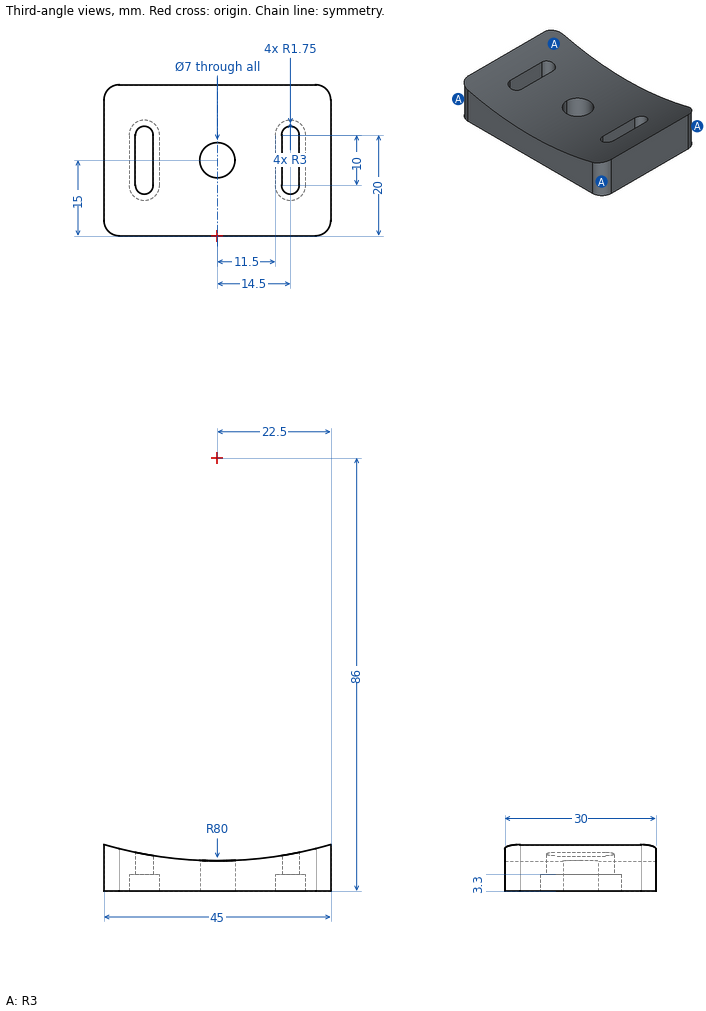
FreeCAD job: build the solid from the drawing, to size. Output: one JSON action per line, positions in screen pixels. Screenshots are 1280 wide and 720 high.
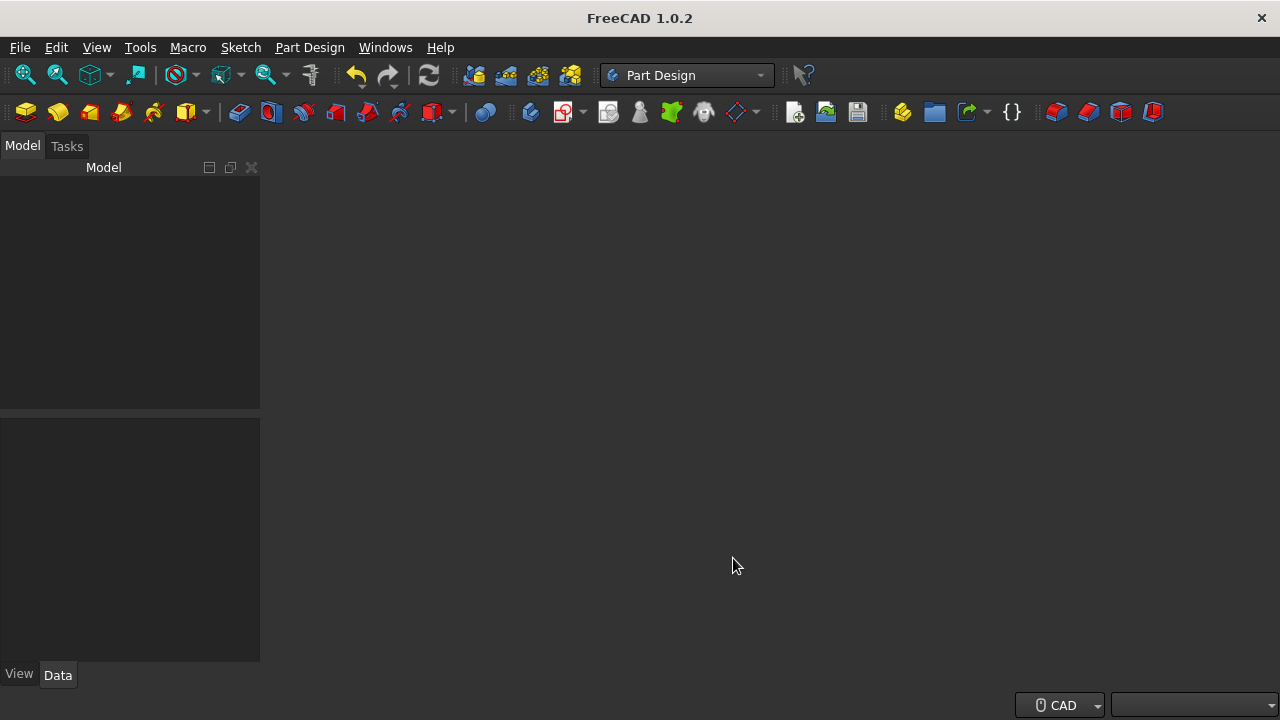
{"action": "key", "text": "ctrl+n"}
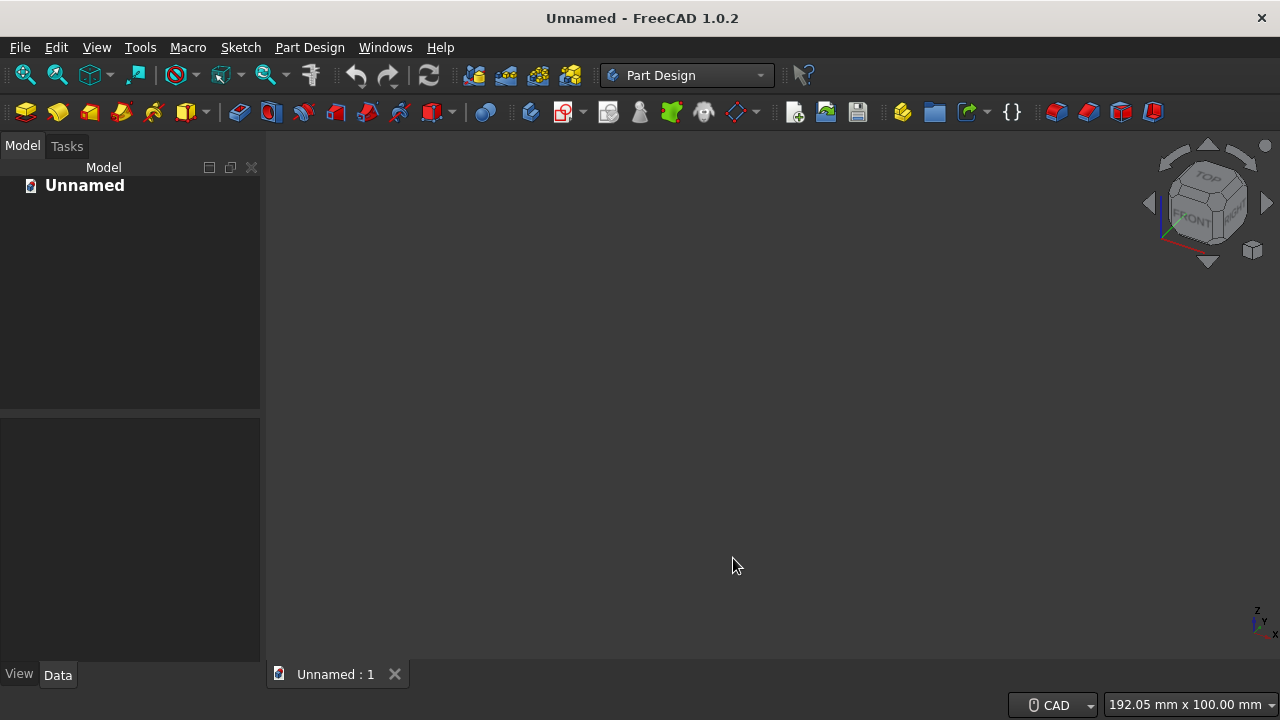
{"action": "left_click", "coordinate": [564, 112]}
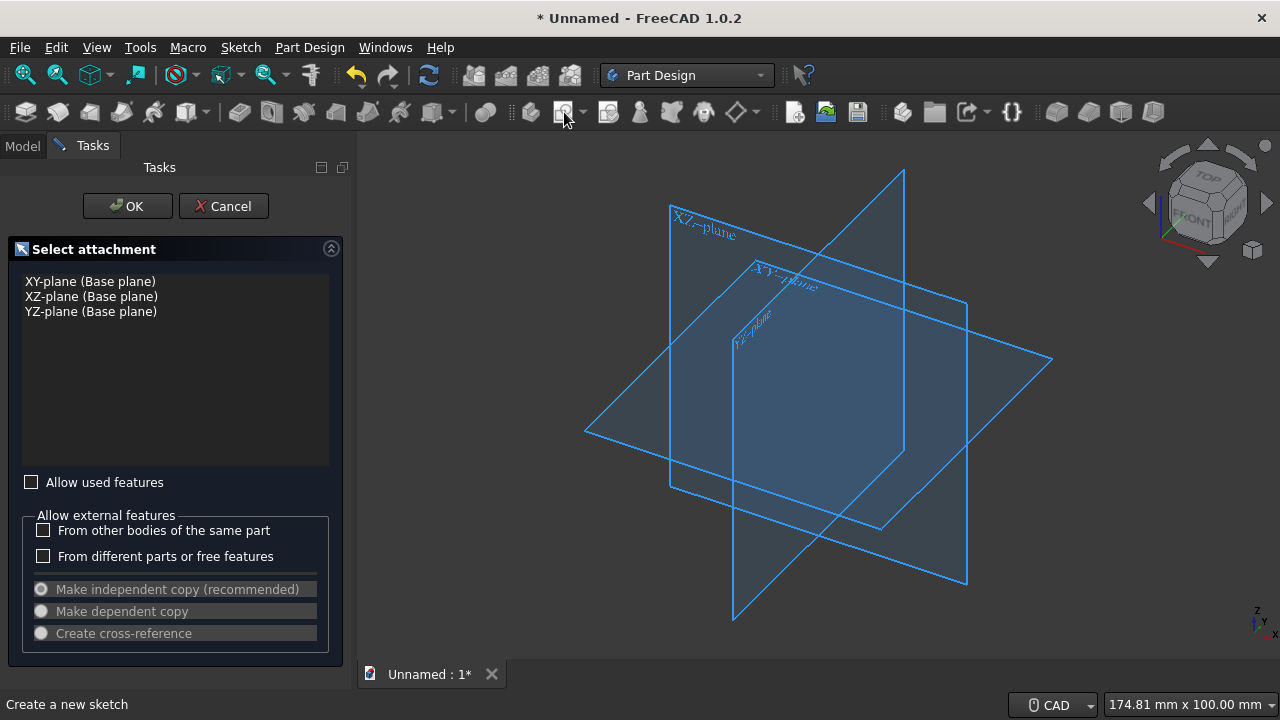
{"action": "left_click", "coordinate": [82, 296]}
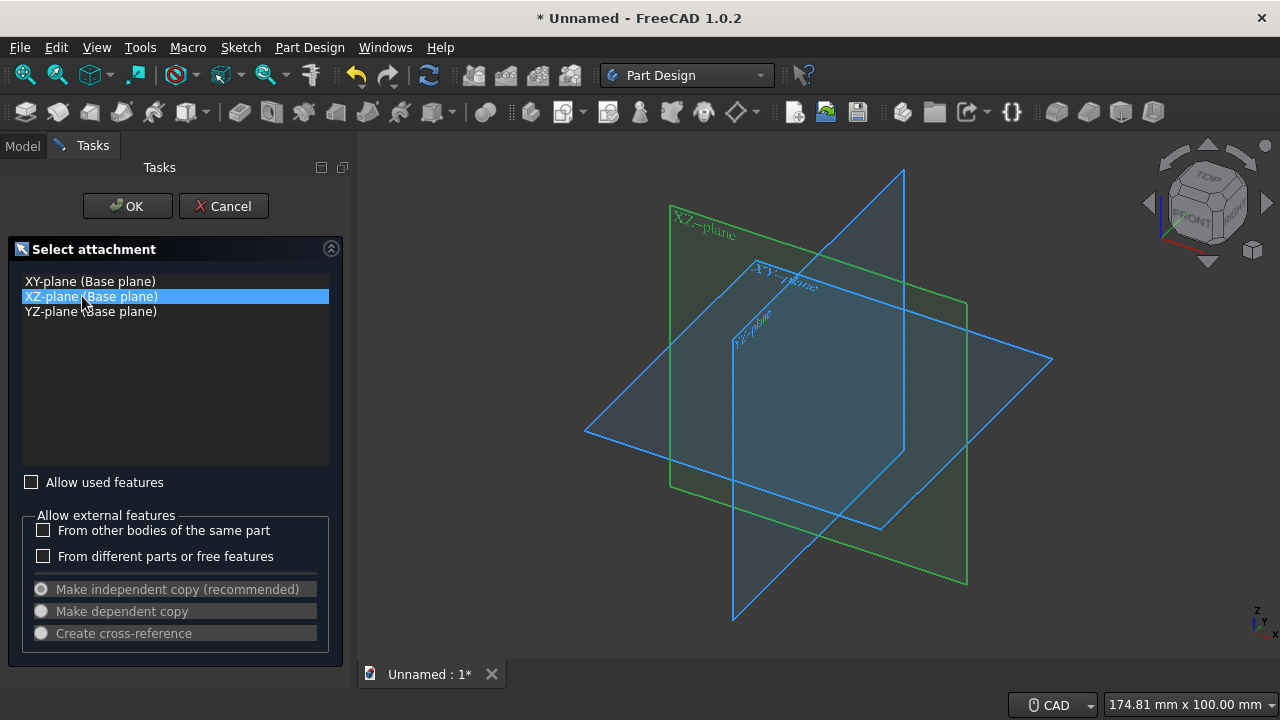
{"action": "left_click", "coordinate": [128, 206]}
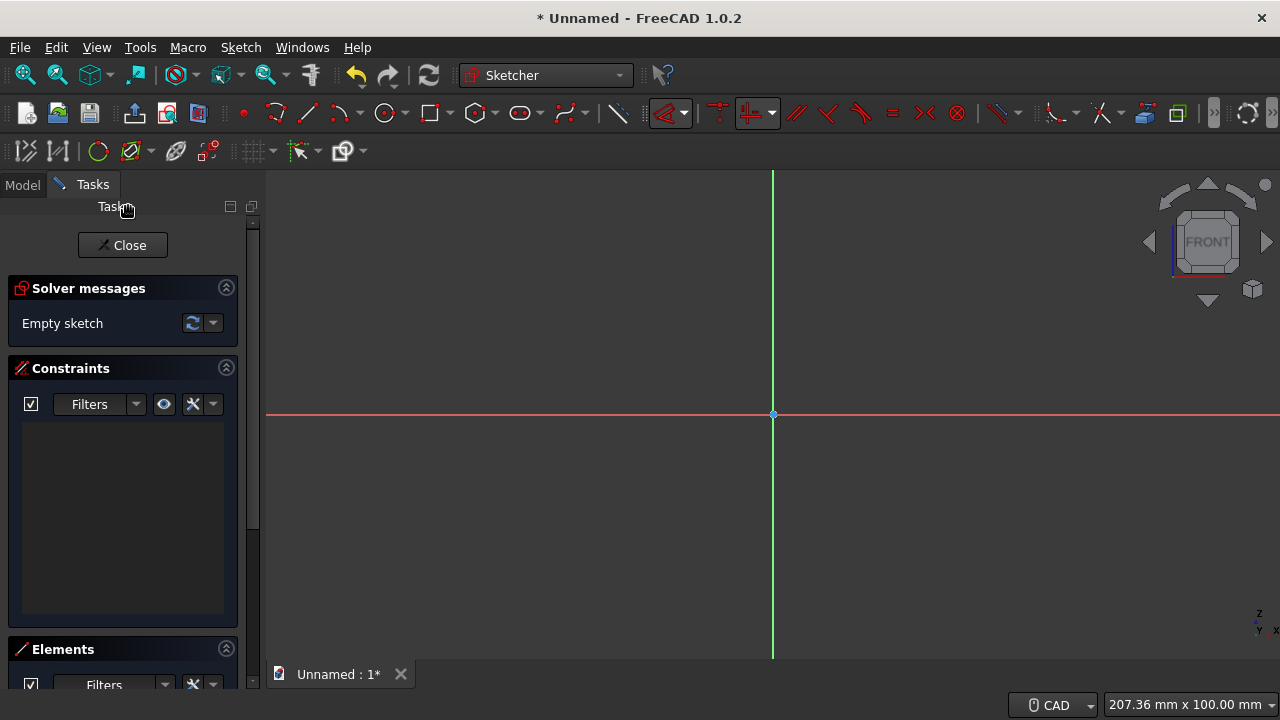
{"action": "scroll", "coordinate": [621, 198], "scroll_direction": "down", "scroll_amount": 3}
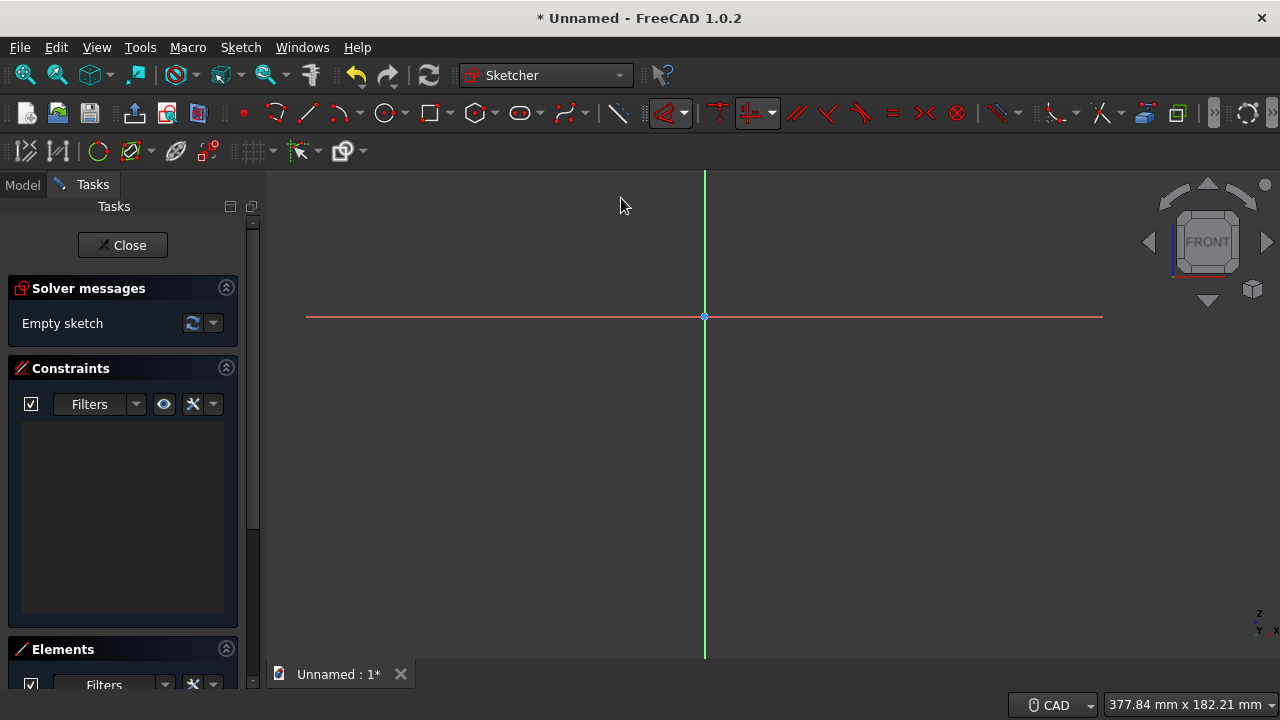
{"action": "left_click", "coordinate": [276, 114]}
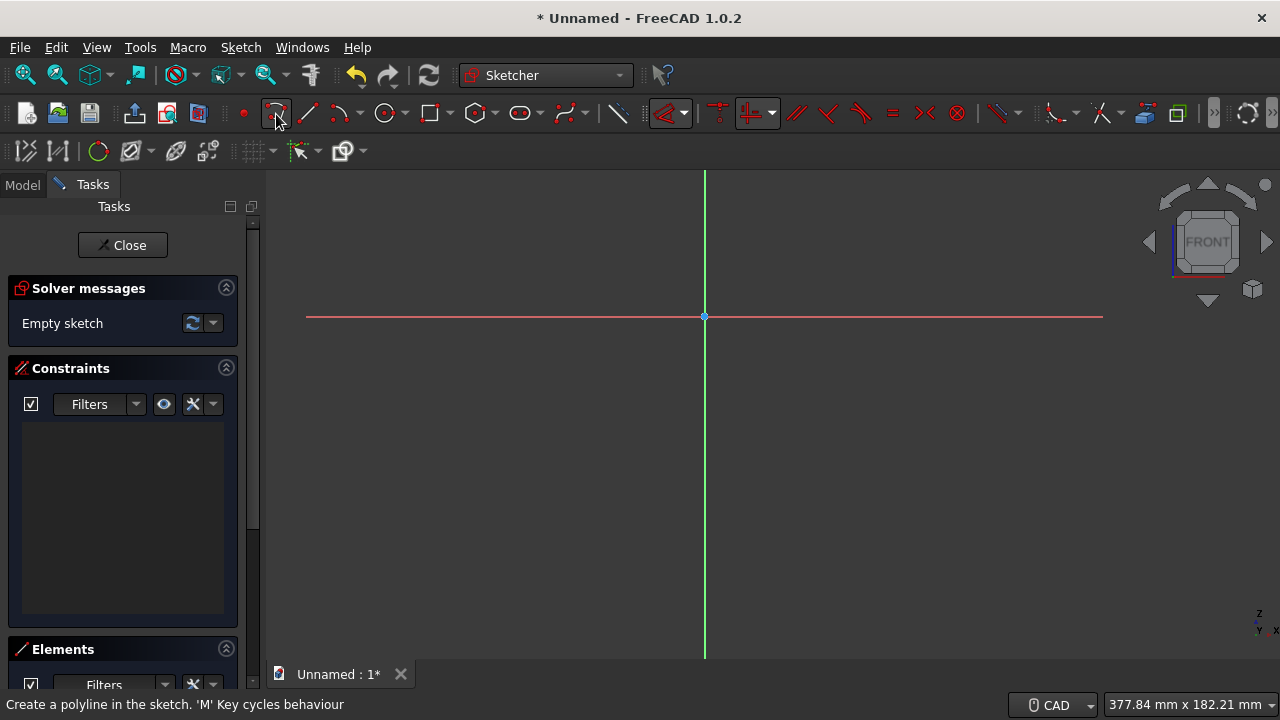
{"action": "left_click", "coordinate": [765, 523]}
{"action": "left_click", "coordinate": [765, 548]}
{"action": "left_click", "coordinate": [644, 548]}
{"action": "left_click", "coordinate": [644, 523]}
{"action": "right_click", "coordinate": [644, 523]}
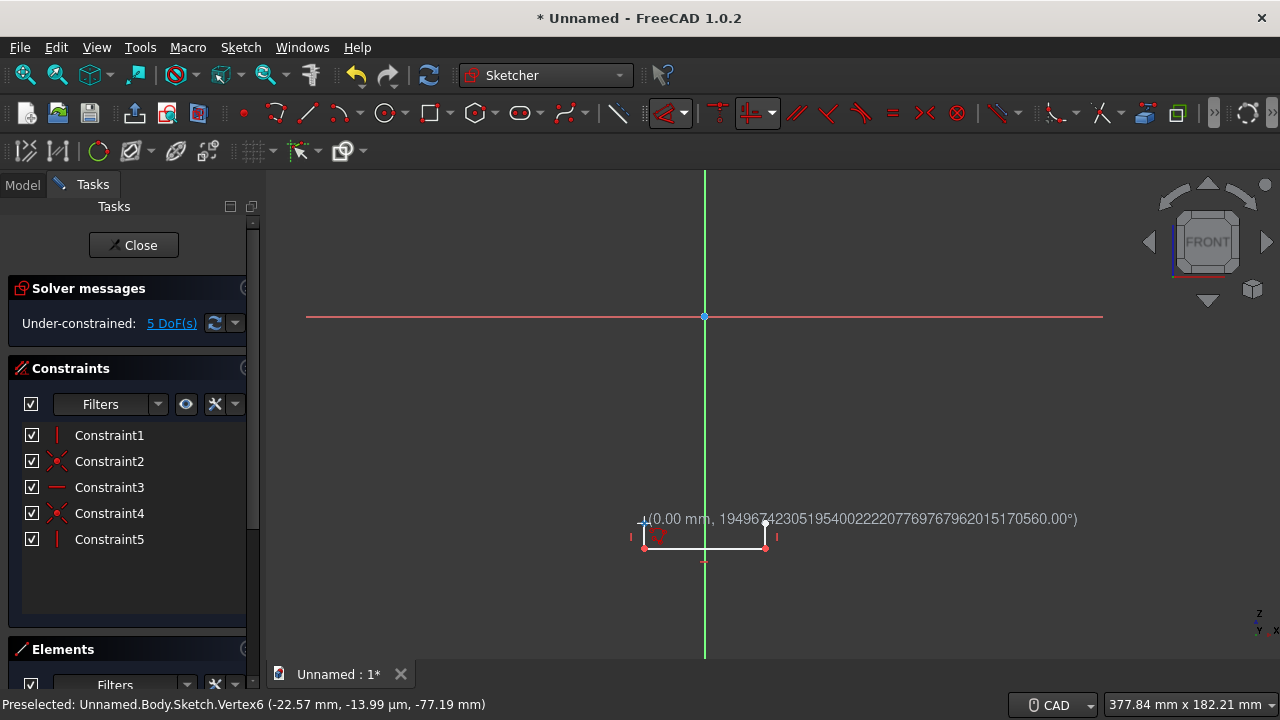
{"action": "key", "text": "g 3 a"}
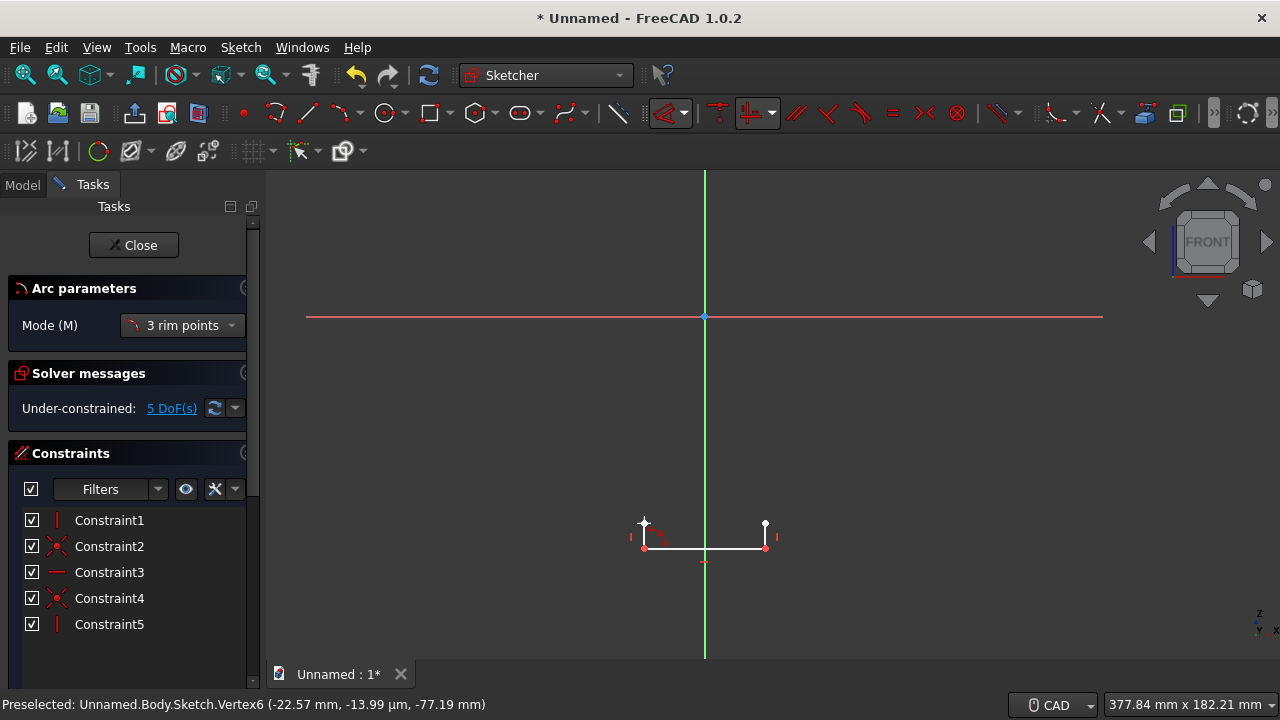
{"action": "scroll", "coordinate": [644, 523], "scroll_direction": "up", "scroll_amount": 2}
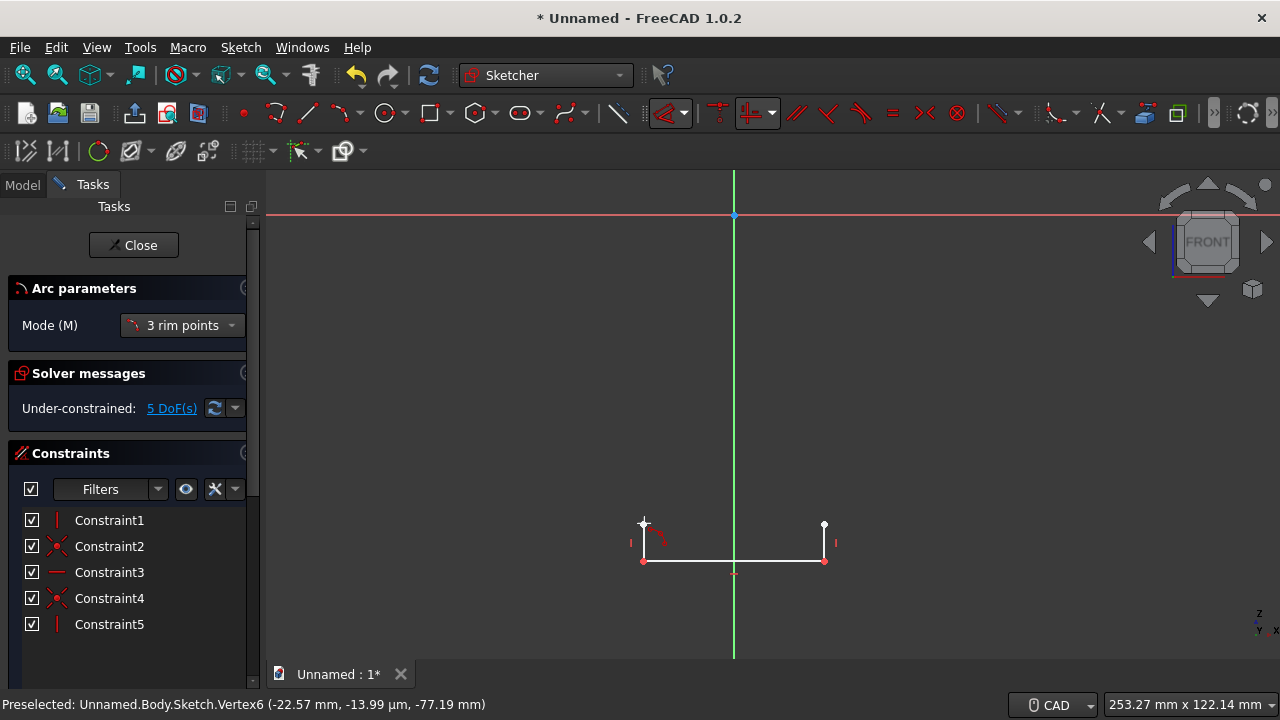
{"action": "left_click", "coordinate": [644, 524]}
{"action": "left_click", "coordinate": [824, 524]}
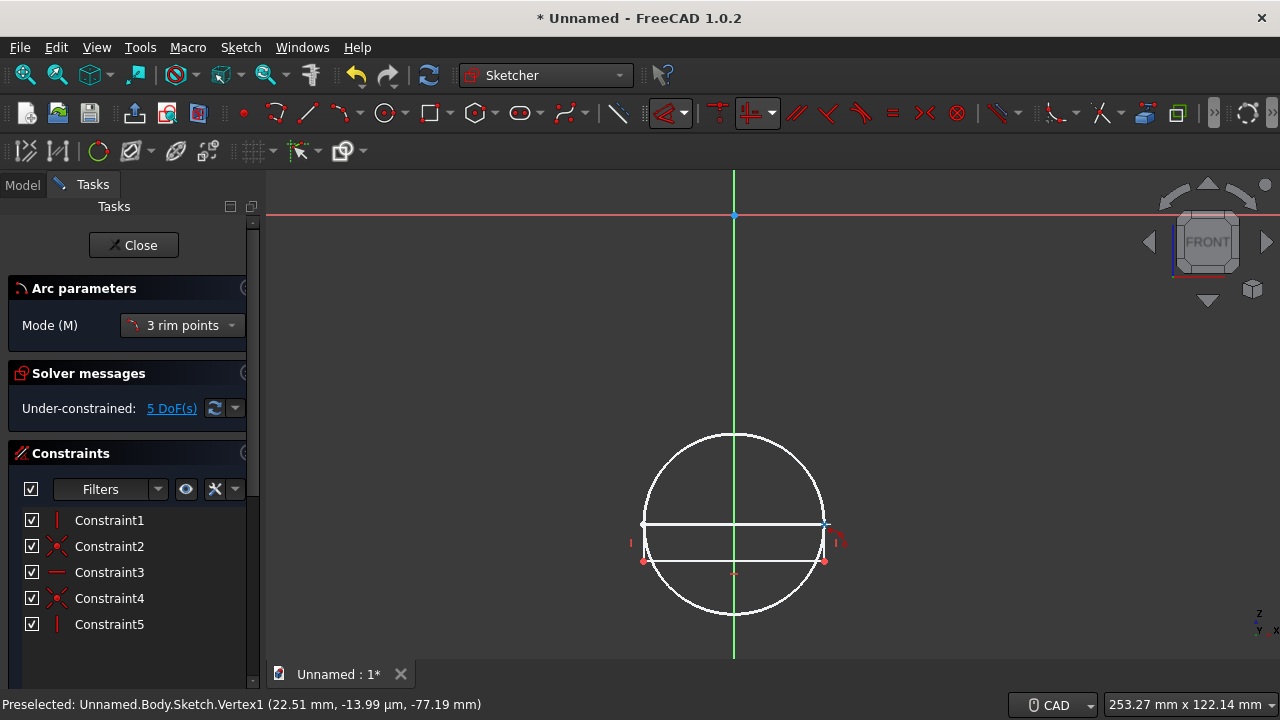
{"action": "scroll", "coordinate": [716, 535], "scroll_direction": "up", "scroll_amount": 2}